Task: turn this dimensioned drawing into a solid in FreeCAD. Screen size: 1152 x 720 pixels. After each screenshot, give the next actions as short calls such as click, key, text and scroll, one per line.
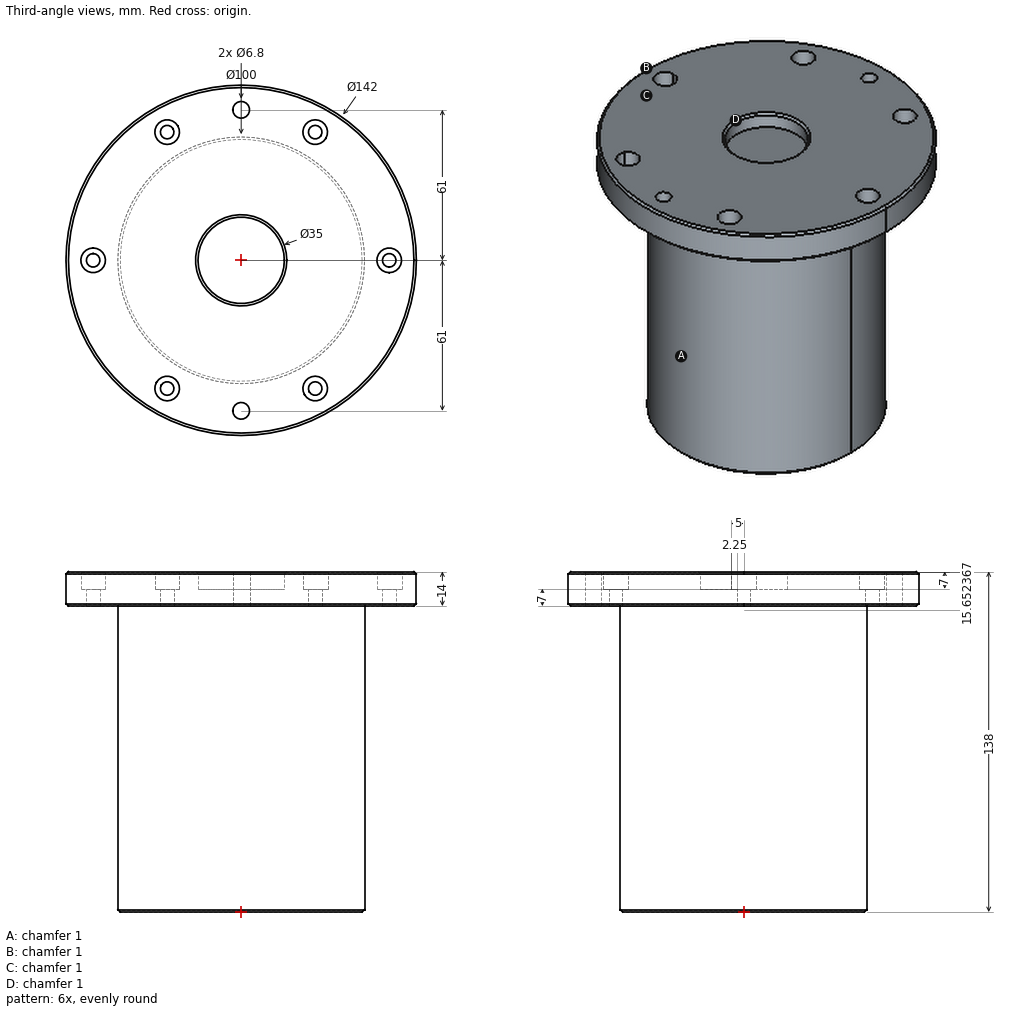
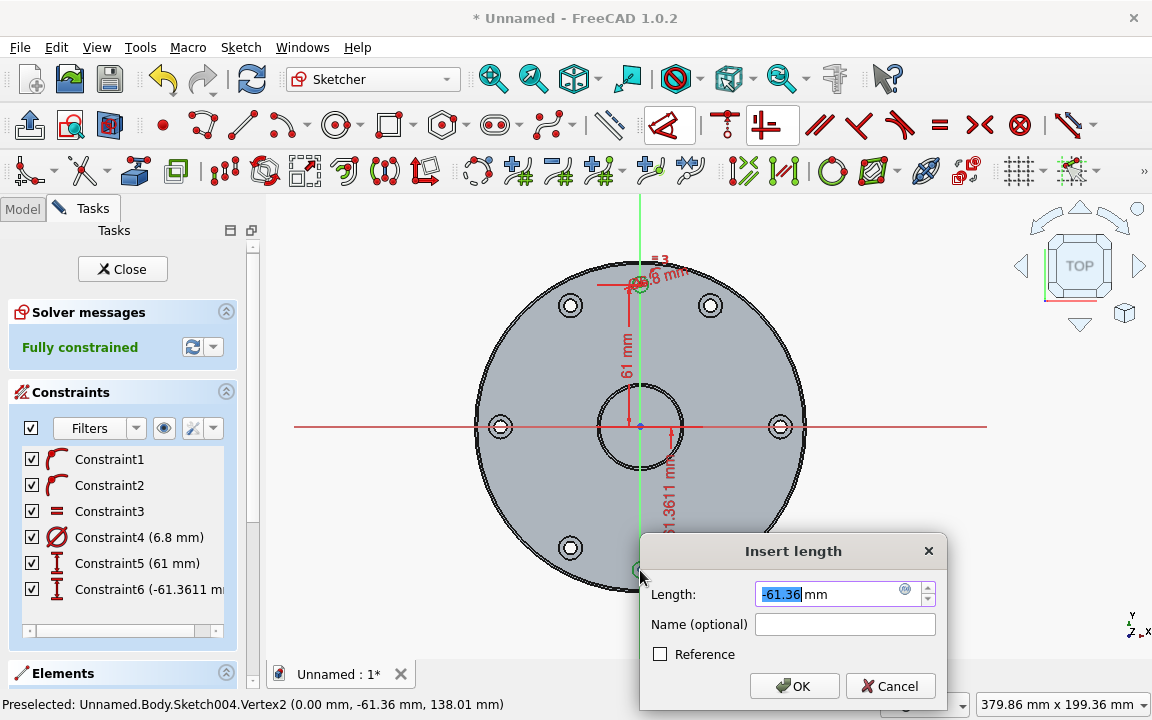
text(-61)
key(Return)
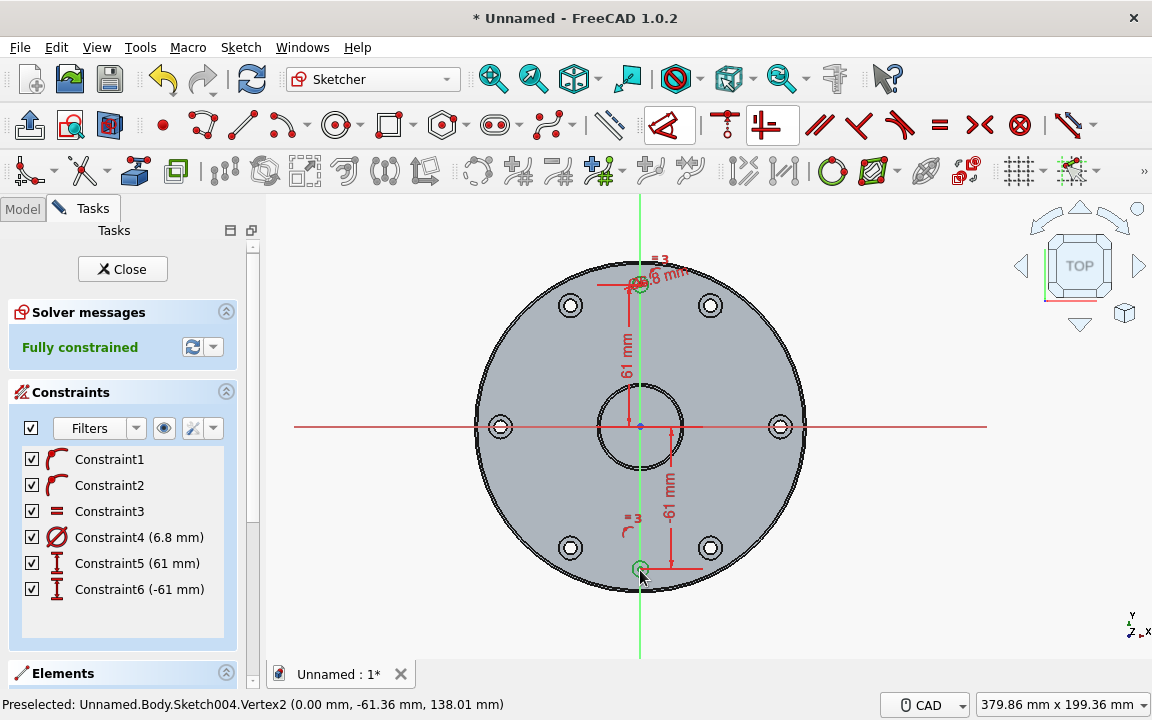
click(123, 269)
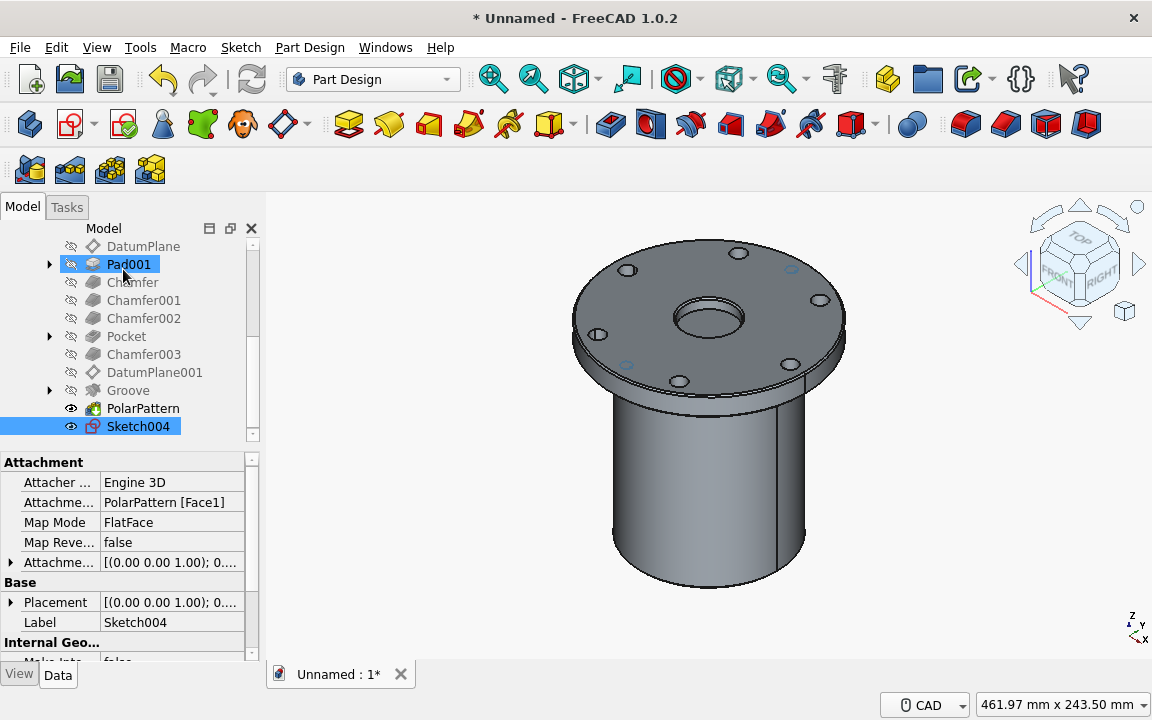
click(612, 124)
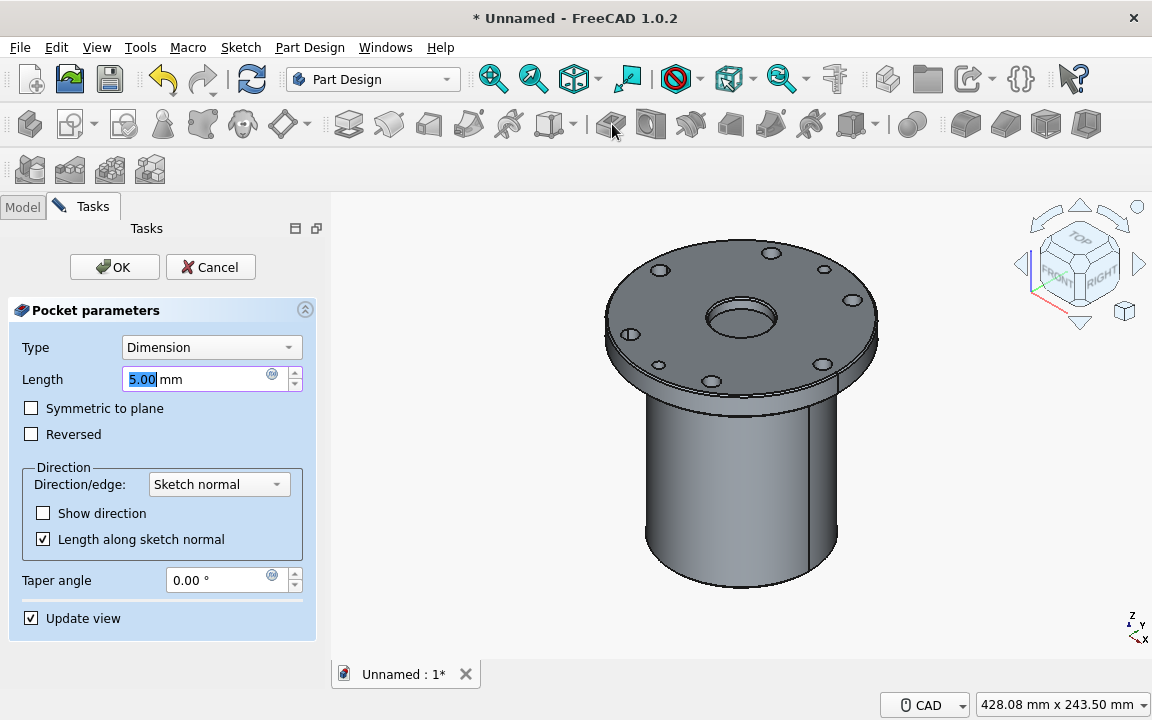
click(212, 348)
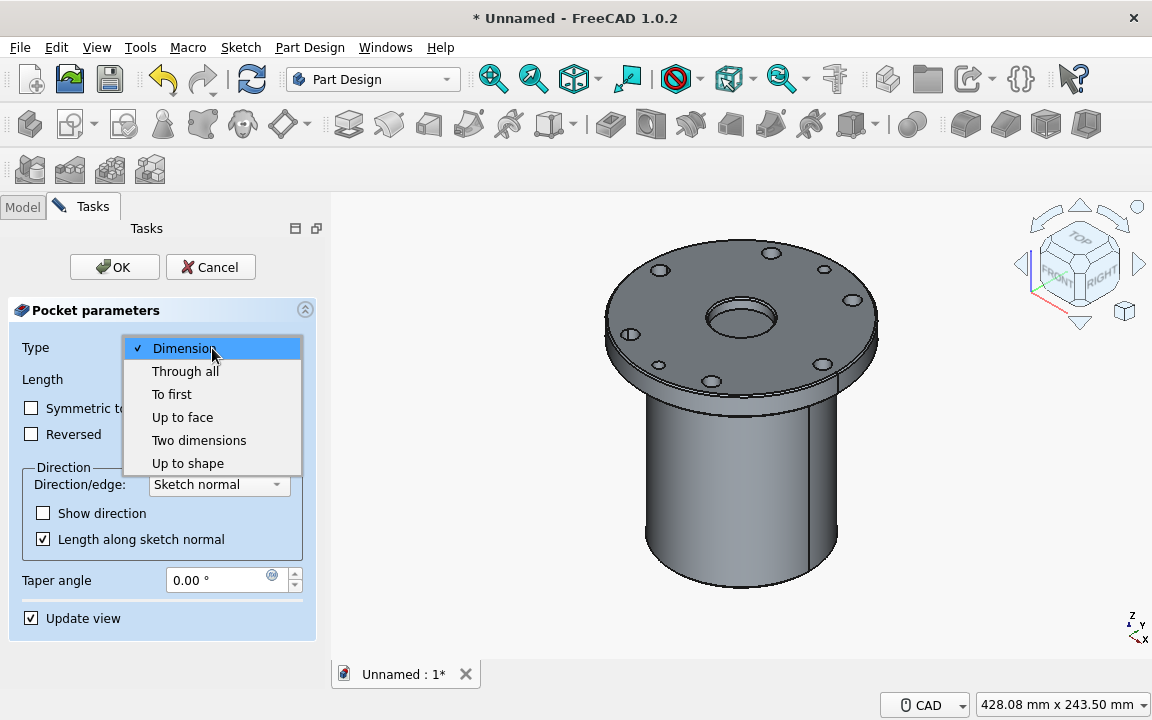
click(212, 372)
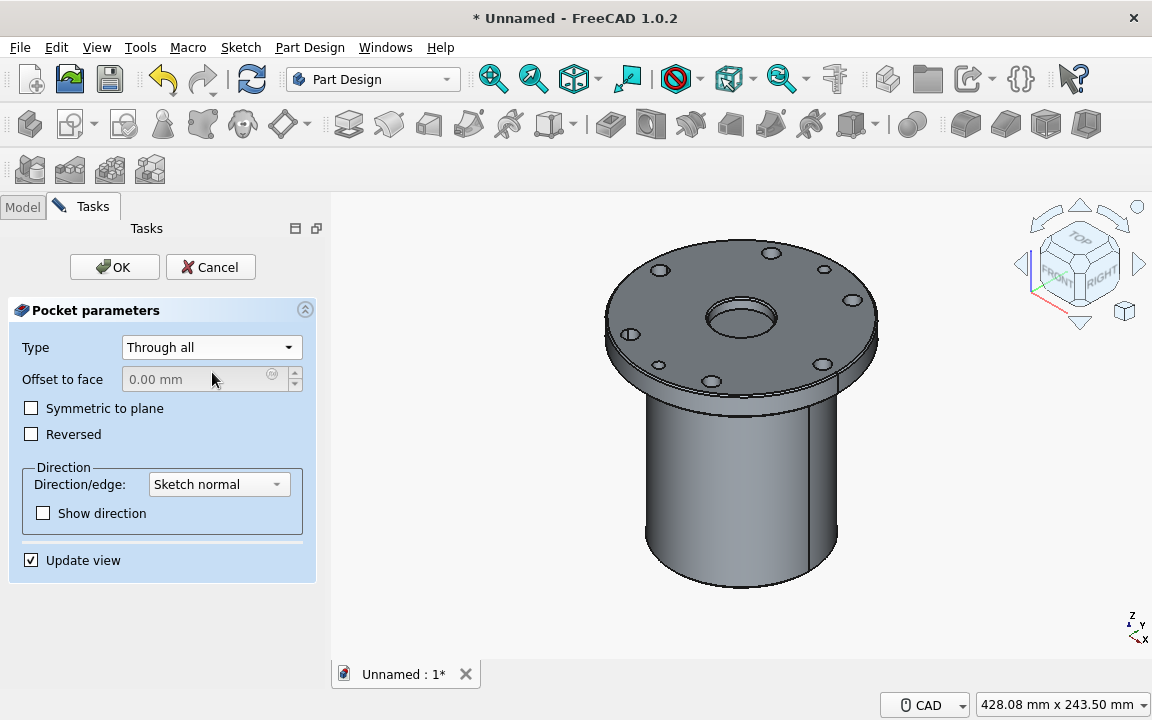
click(115, 267)